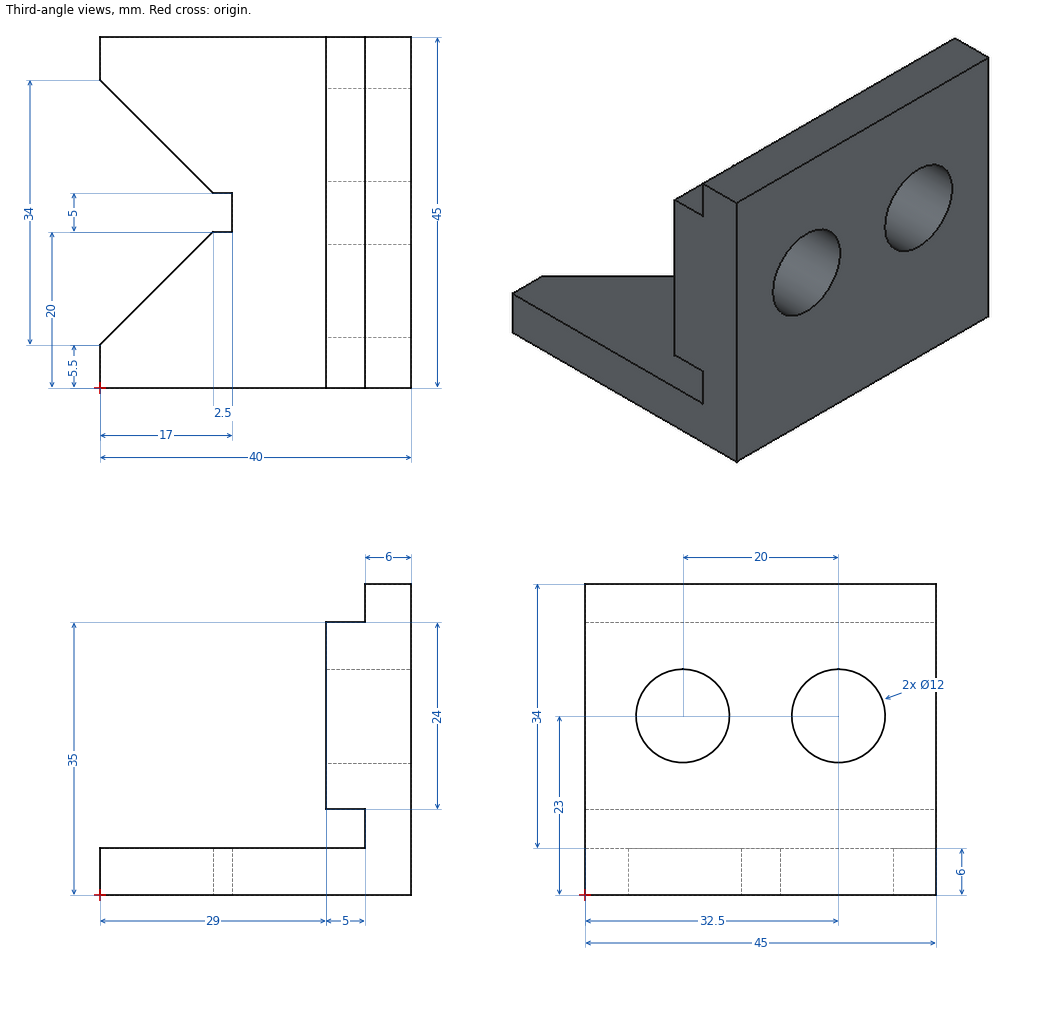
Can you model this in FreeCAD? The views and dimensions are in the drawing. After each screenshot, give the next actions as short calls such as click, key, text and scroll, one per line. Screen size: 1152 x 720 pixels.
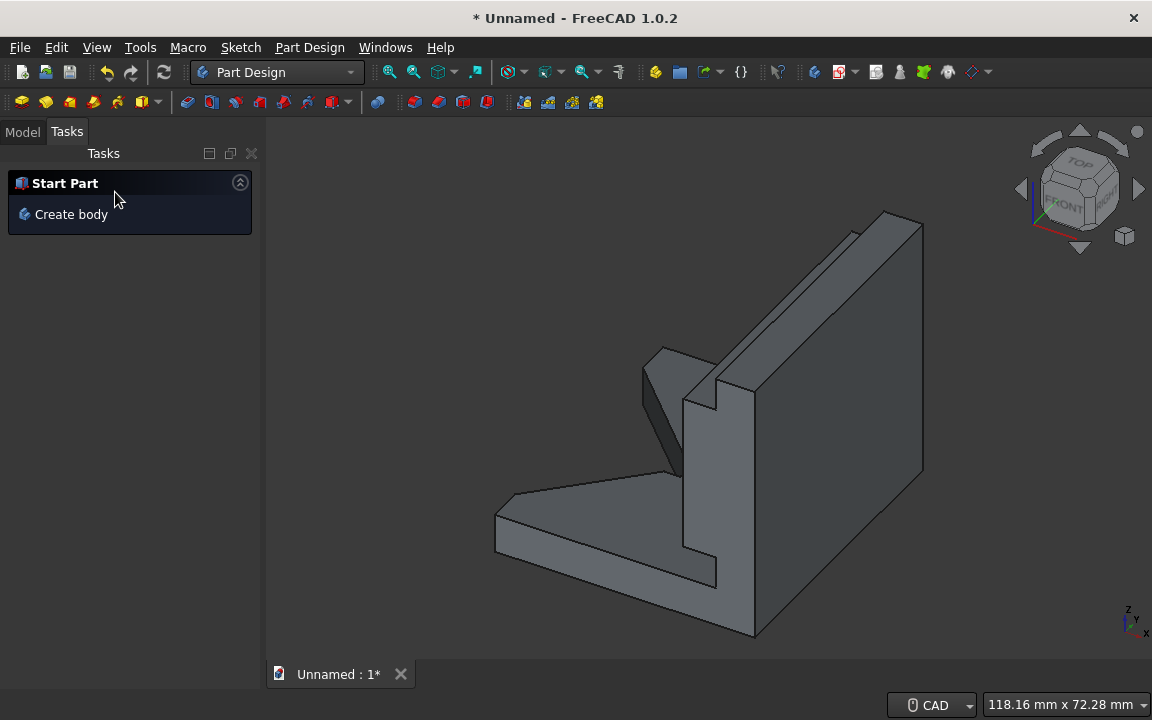
key(6)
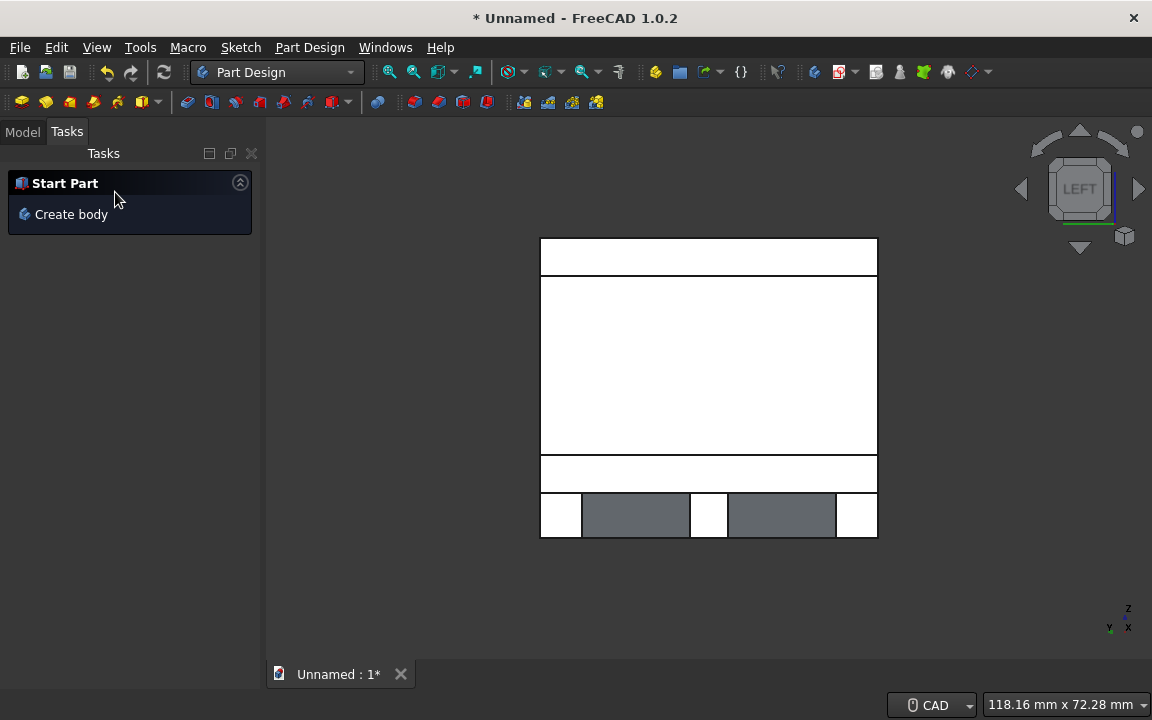
click(661, 365)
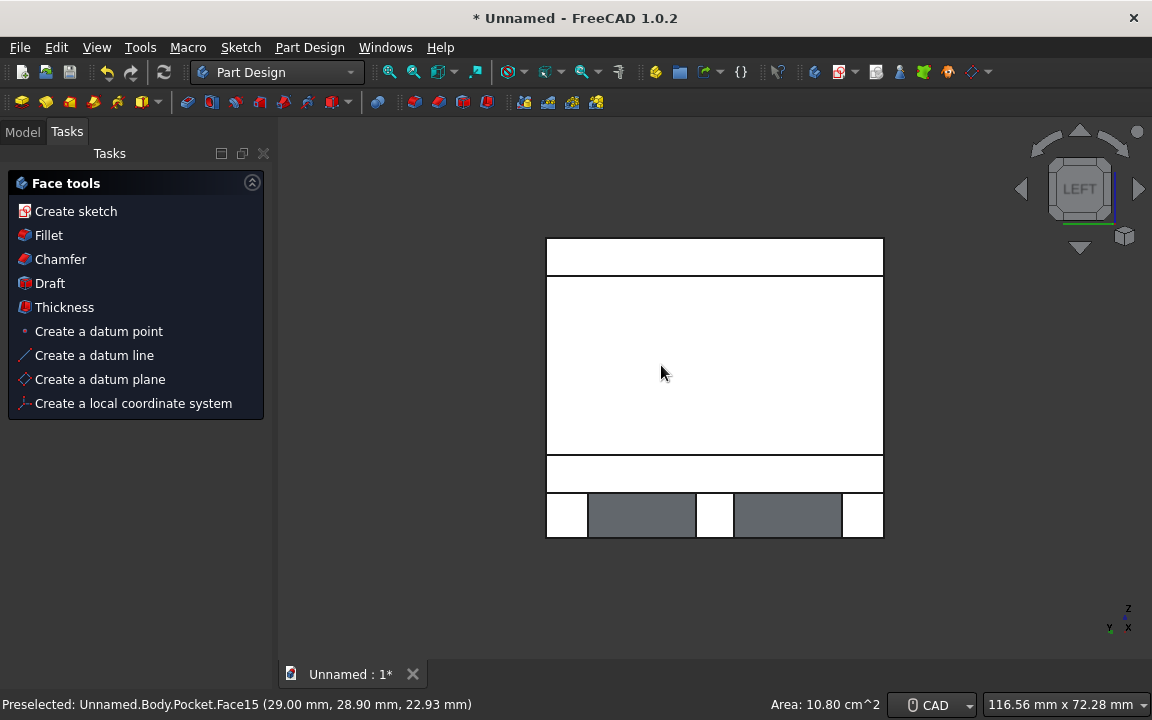
click(840, 72)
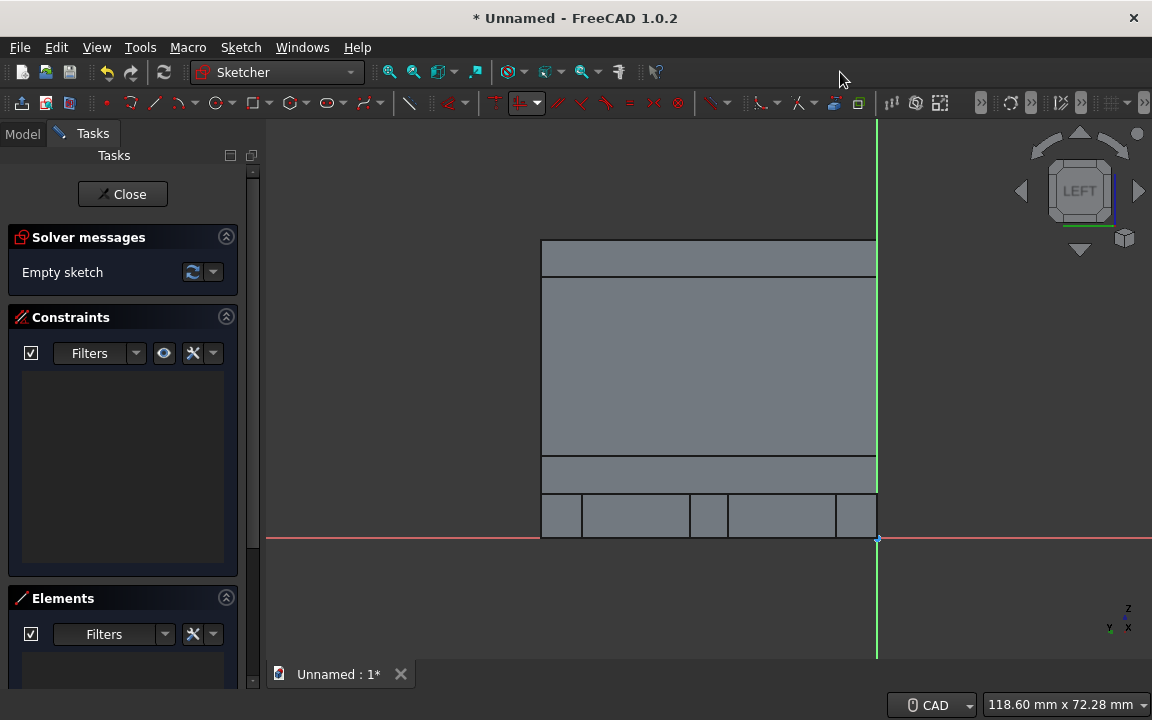
click(70, 104)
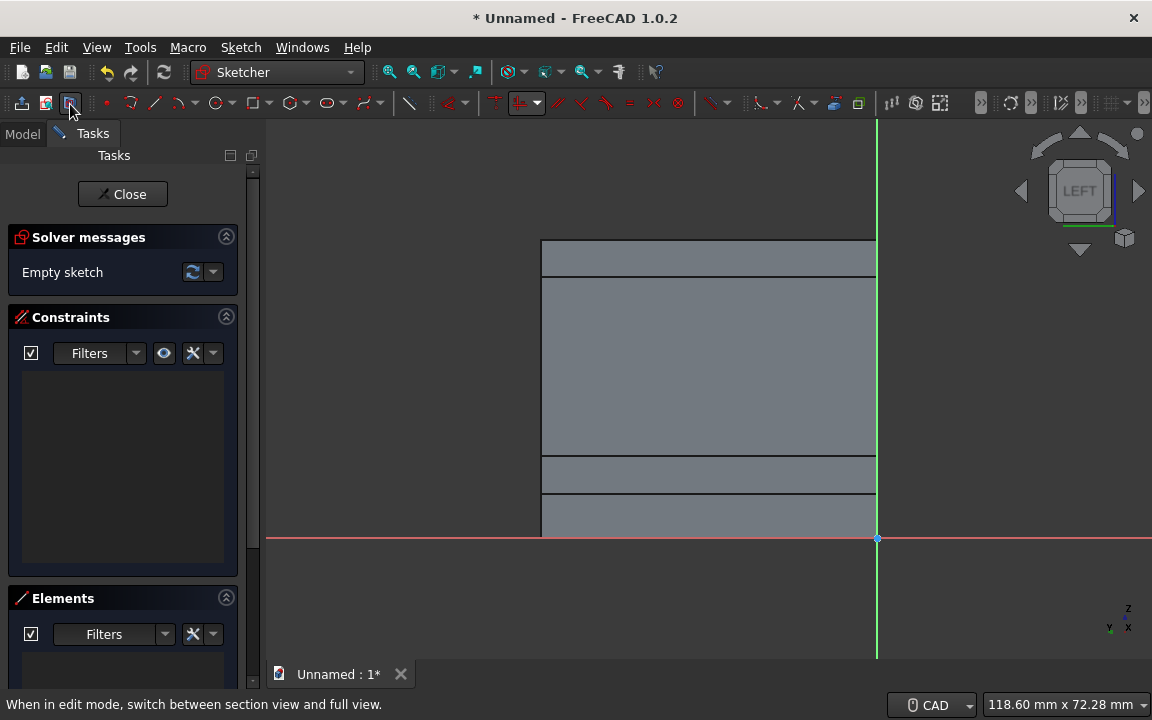
scroll(922, 514, up, 2)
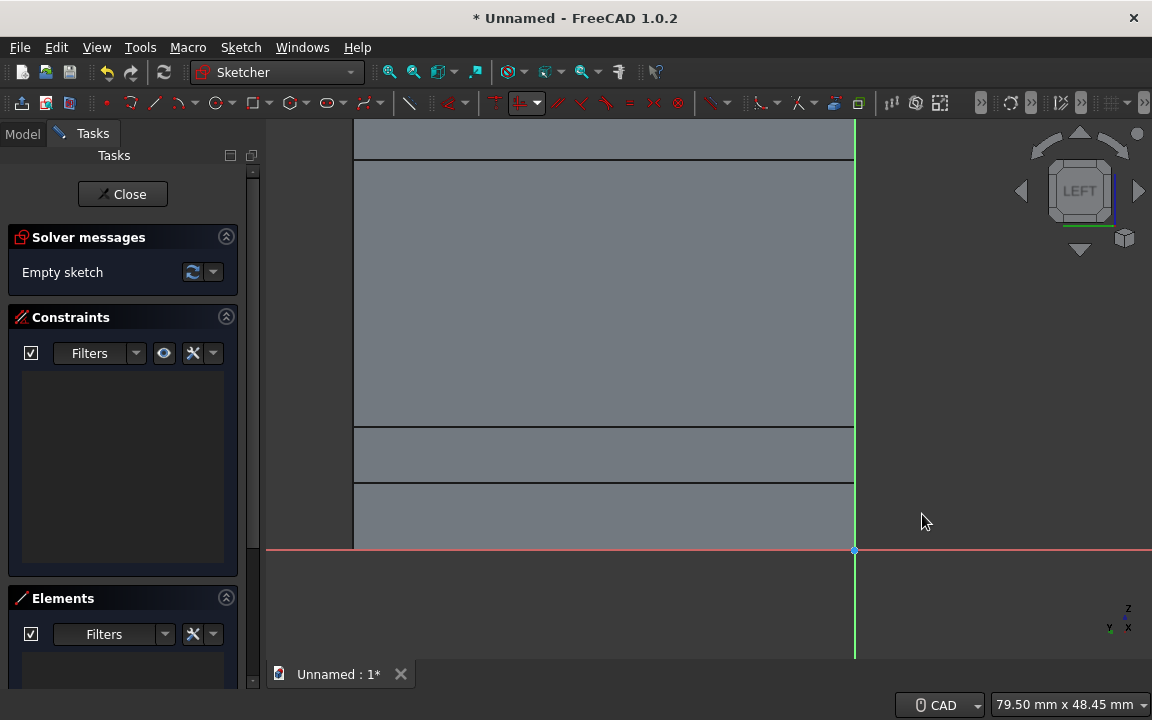
click(216, 104)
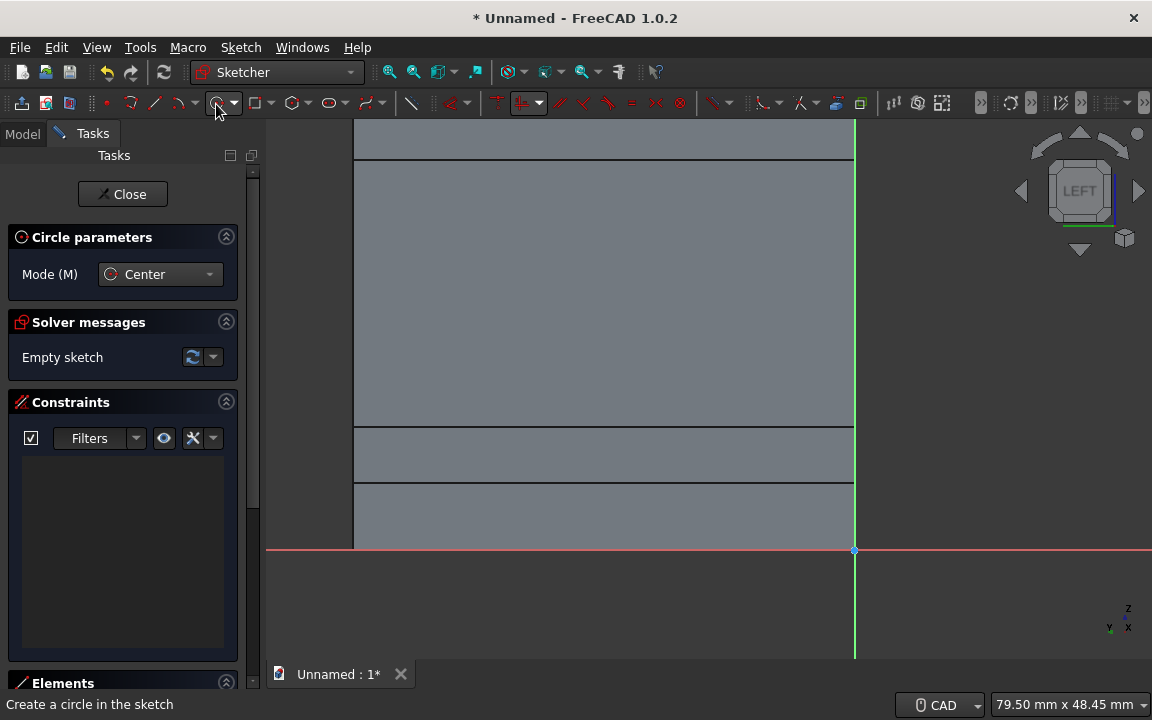
click(492, 294)
click(540, 246)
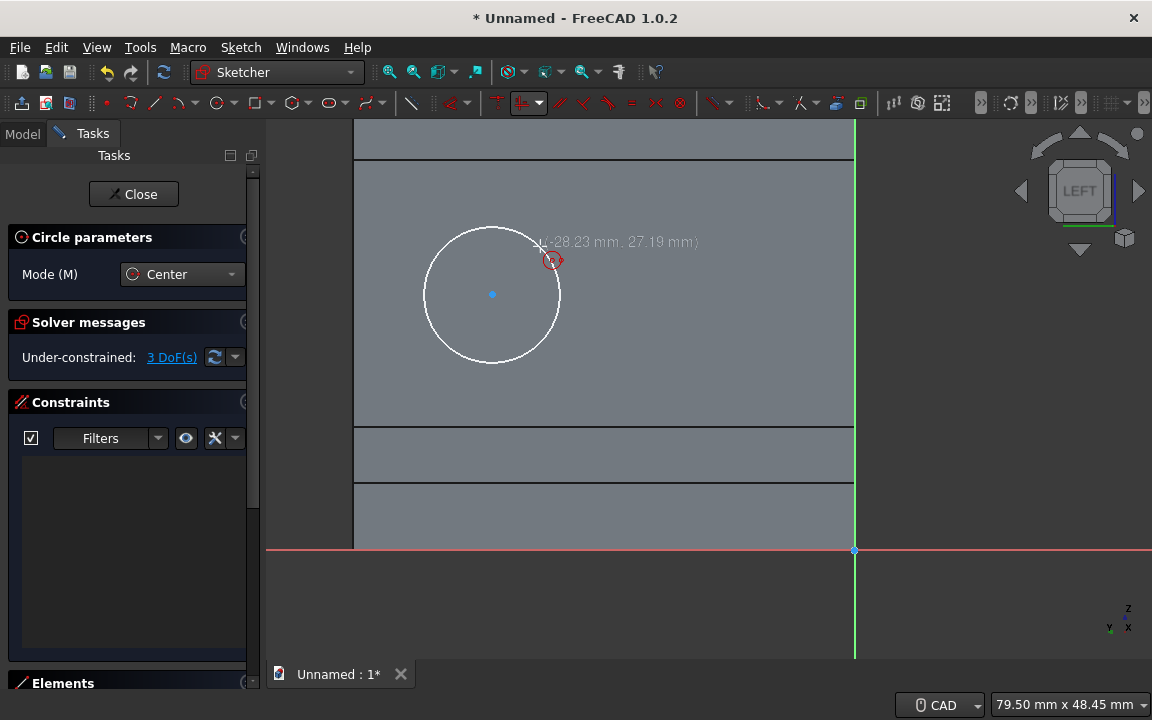
click(715, 294)
click(763, 246)
key(Escape)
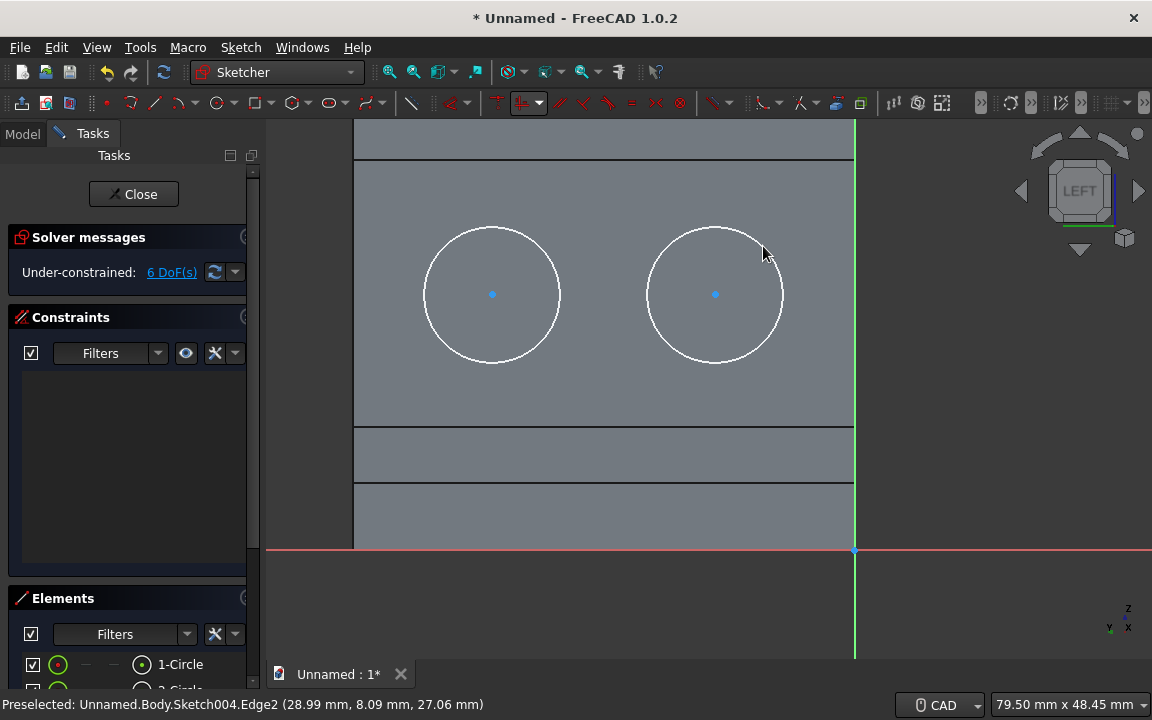
click(540, 247)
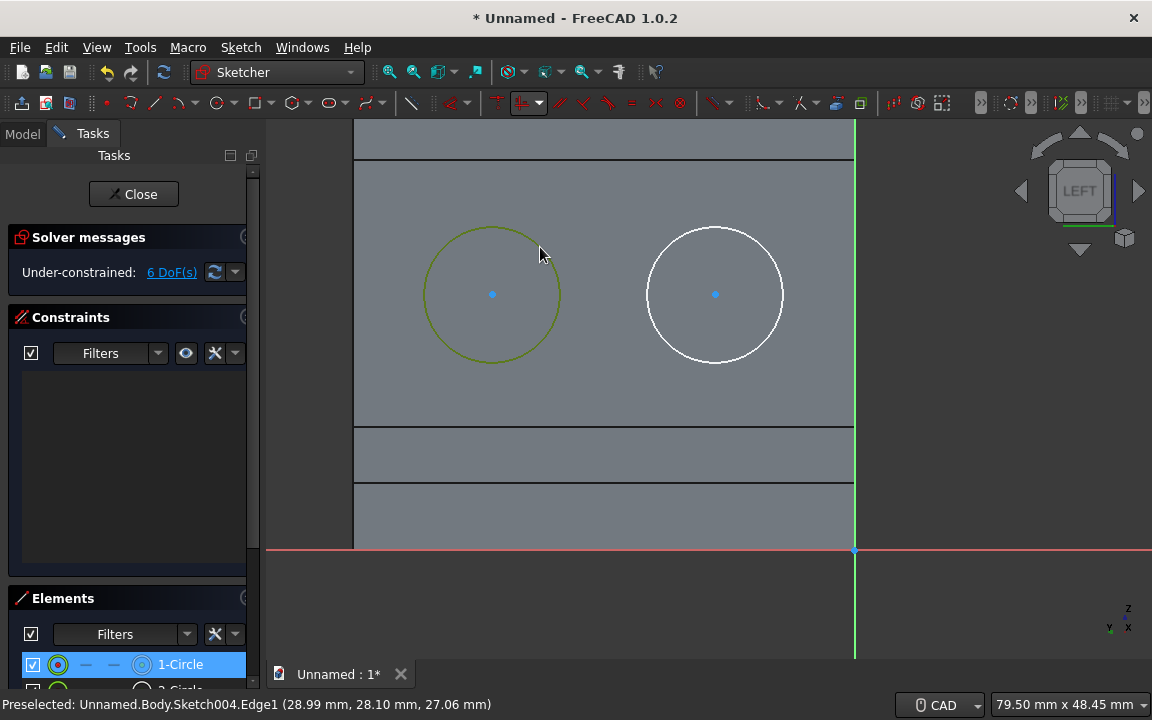
click(763, 247)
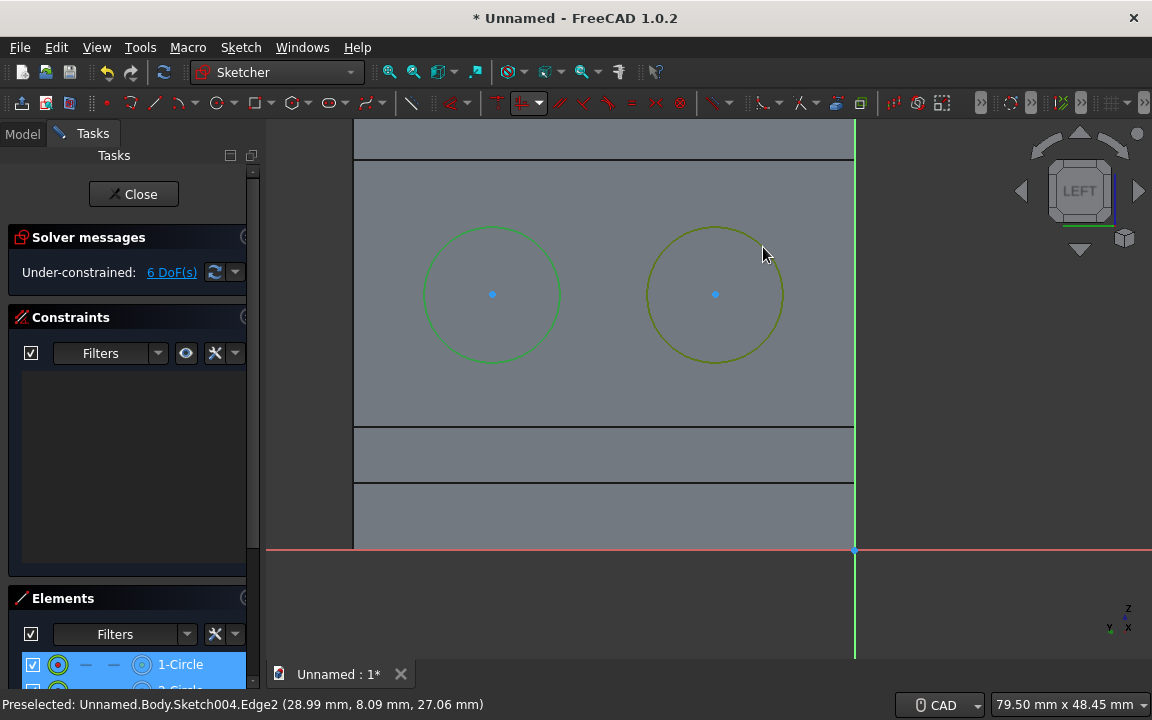
click(632, 104)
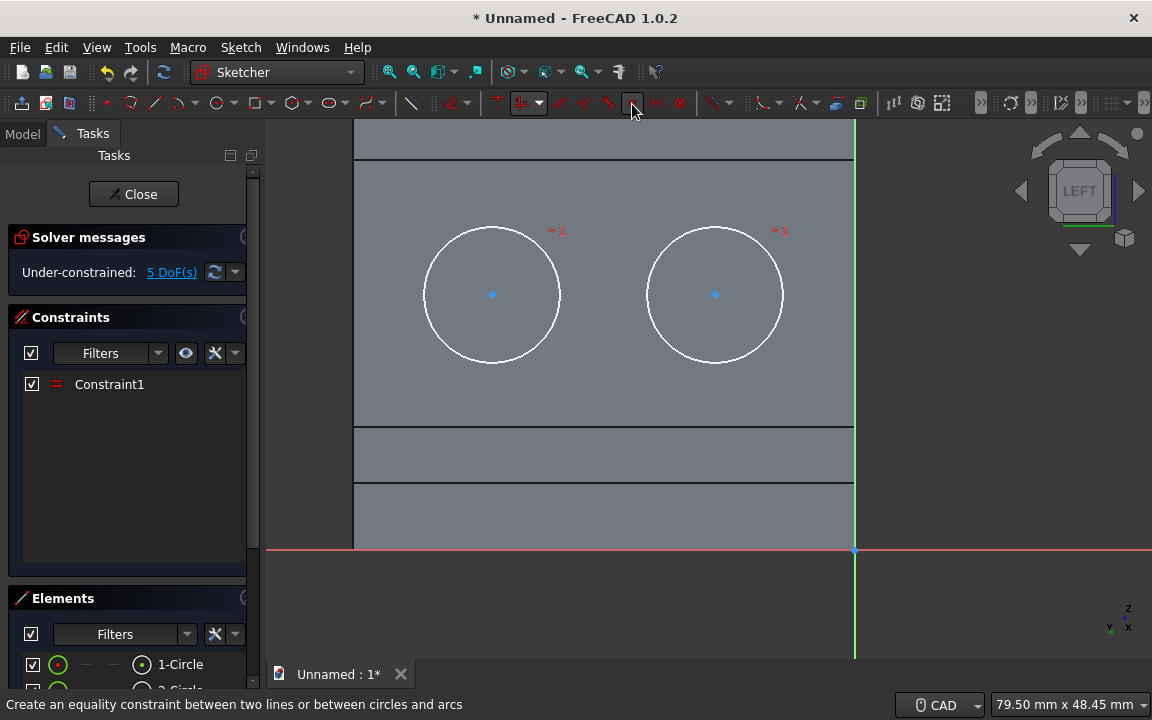
click(492, 295)